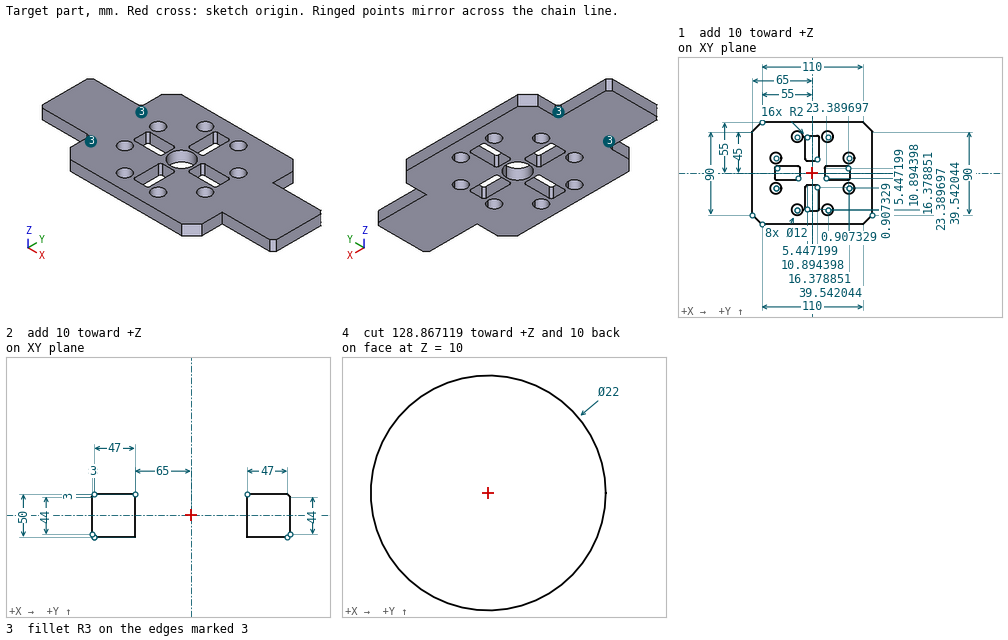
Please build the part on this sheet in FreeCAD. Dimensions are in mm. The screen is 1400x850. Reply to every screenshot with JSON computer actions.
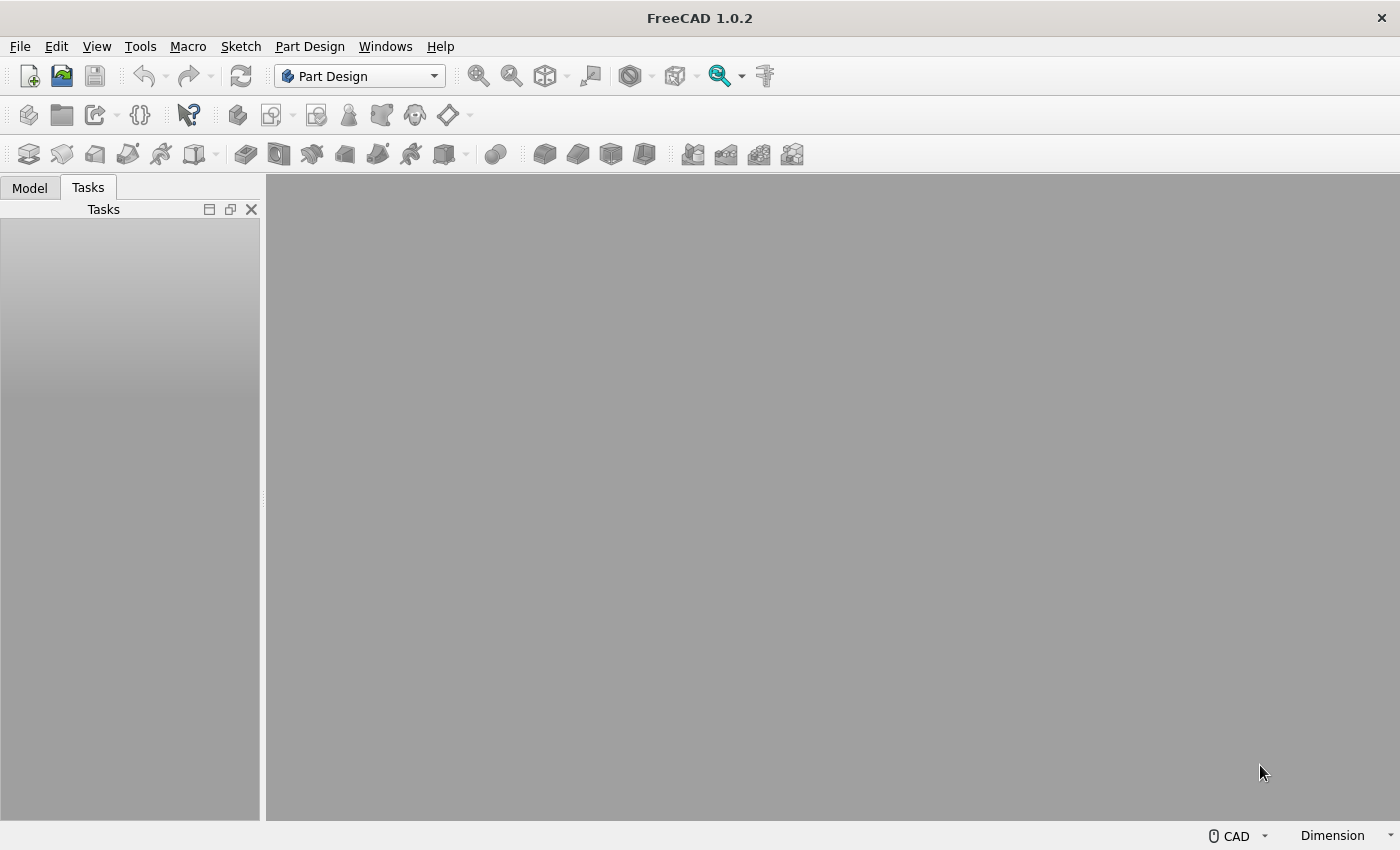
{"action": "left_click", "coordinate": [29, 76]}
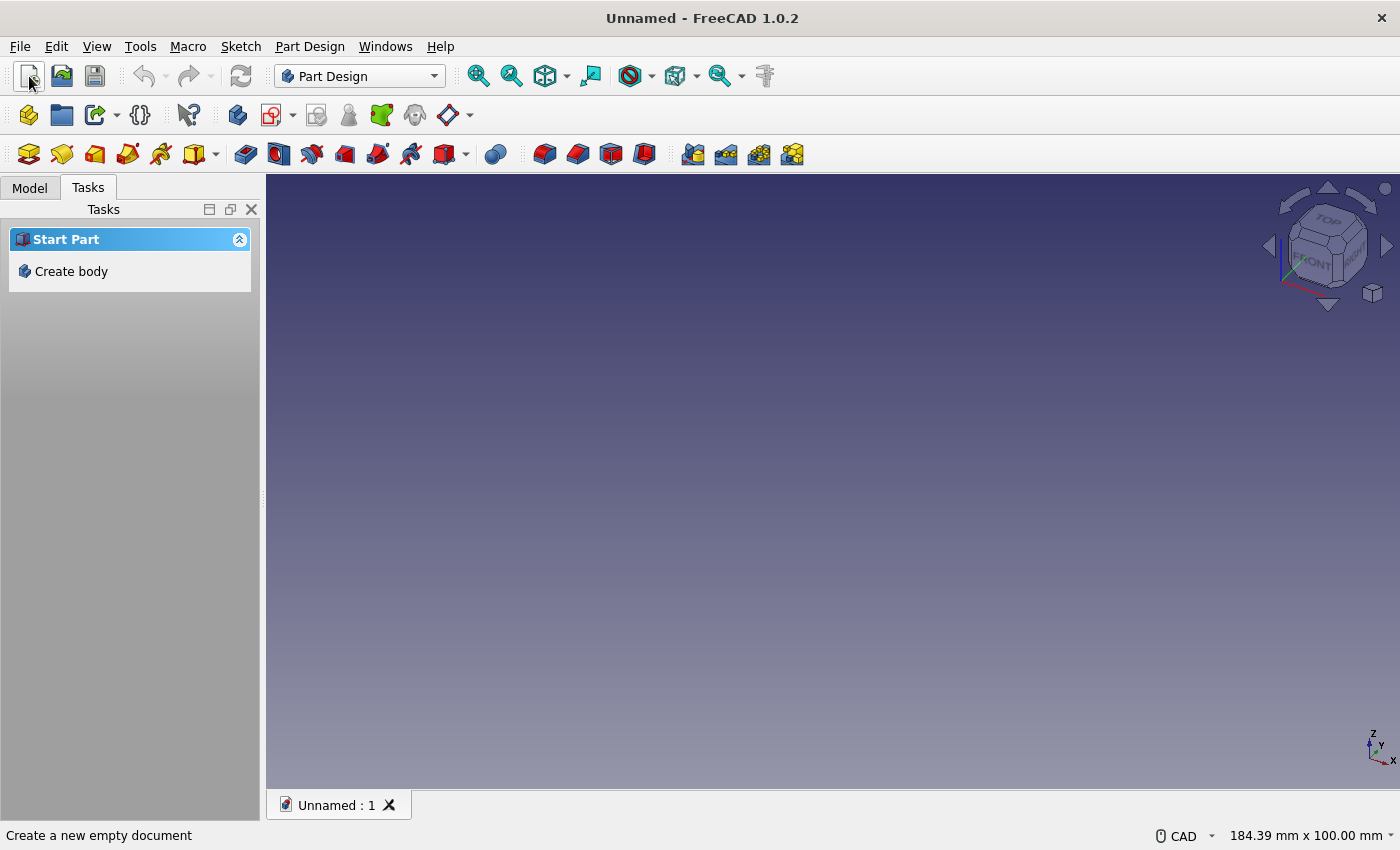
{"action": "left_click", "coordinate": [270, 116]}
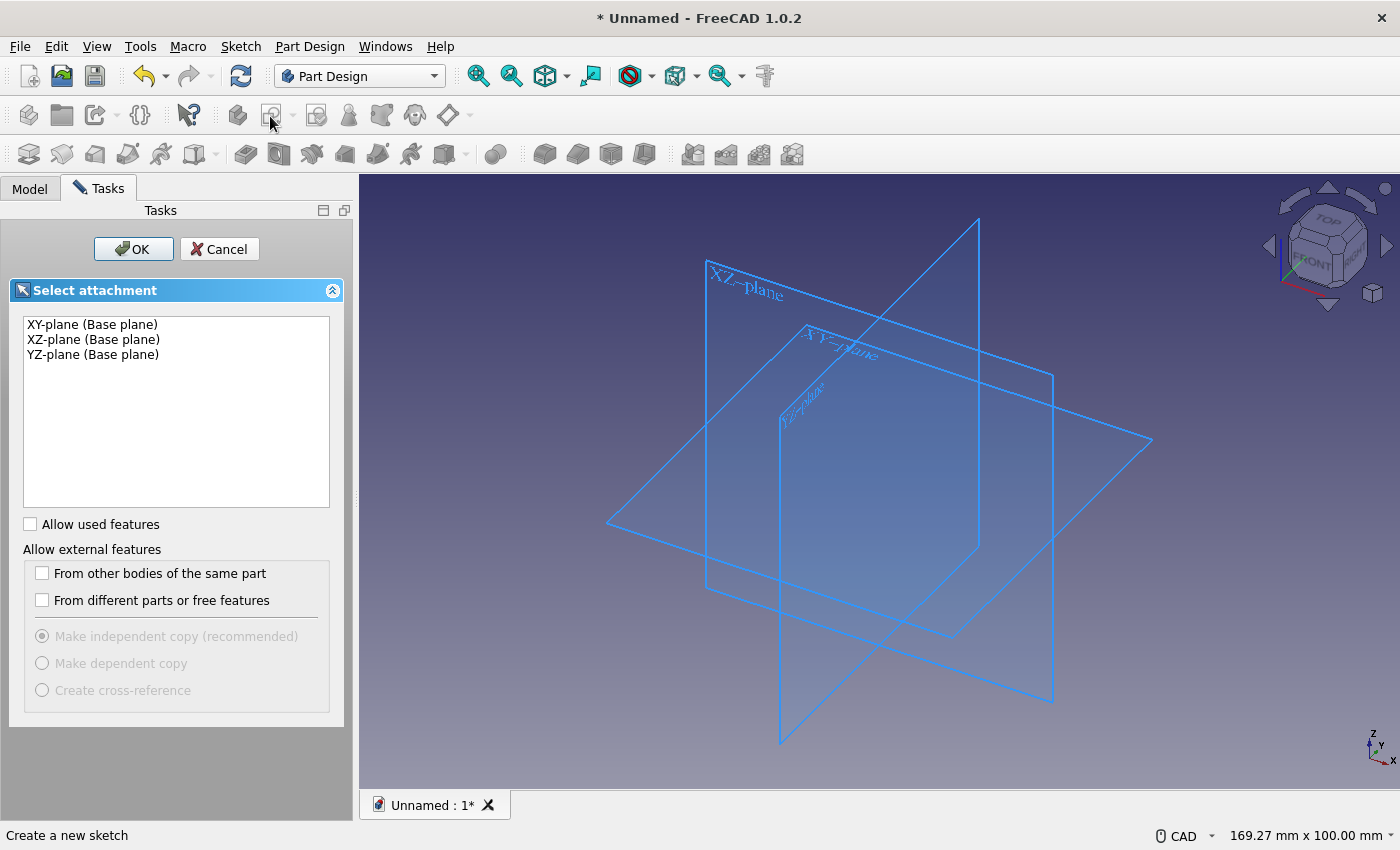
{"action": "left_click", "coordinate": [84, 324]}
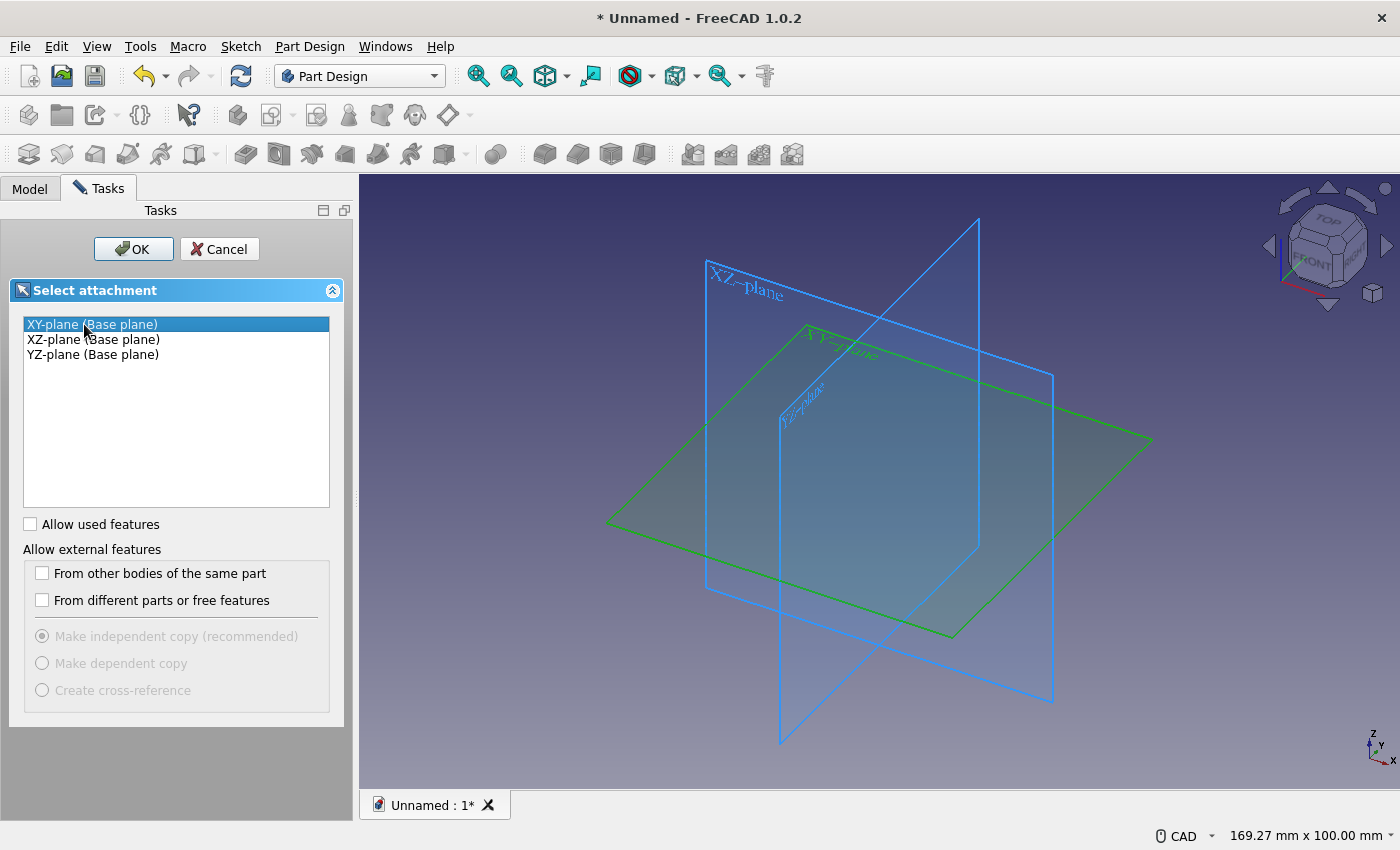
{"action": "left_click", "coordinate": [134, 249]}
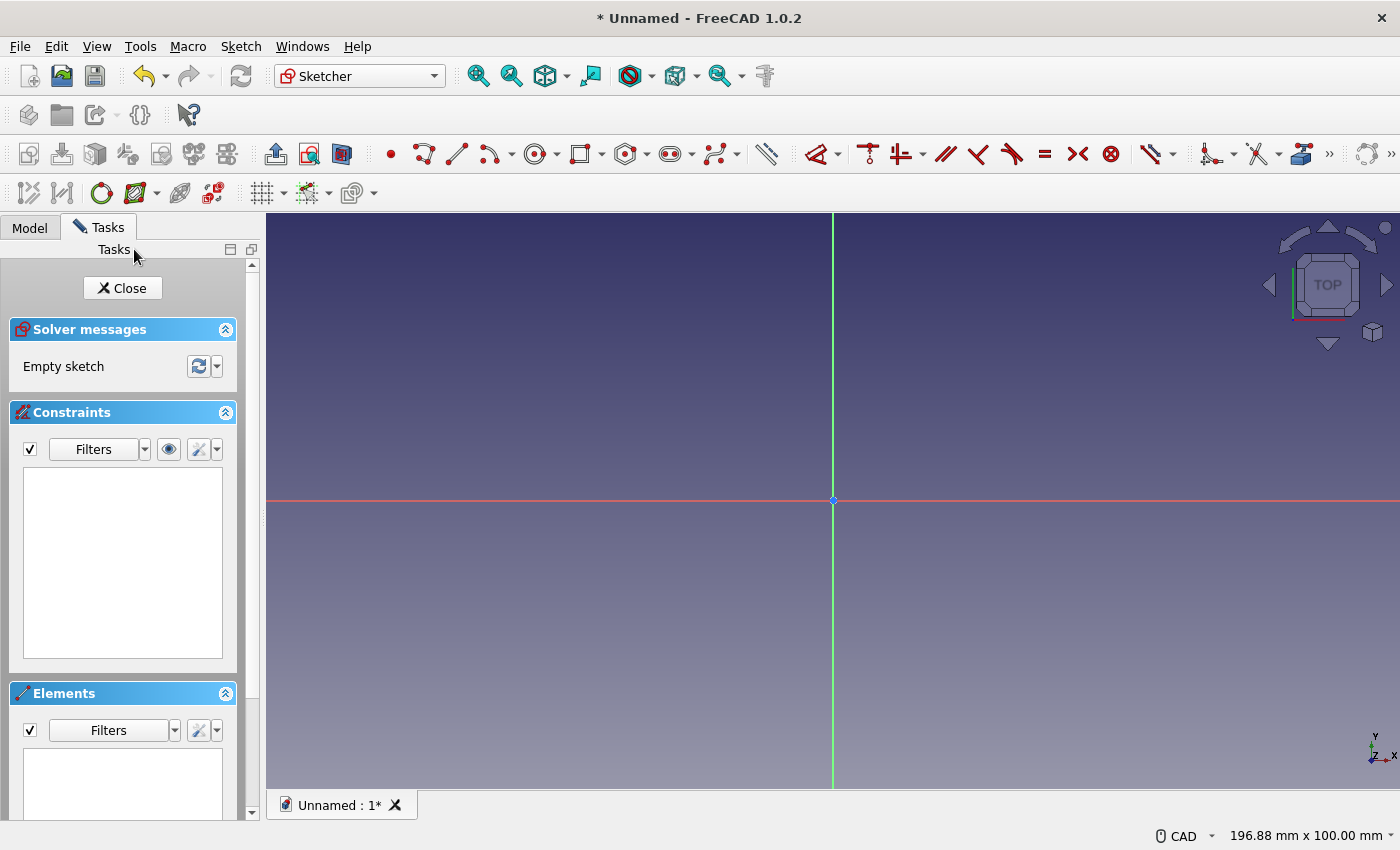
{"action": "scroll", "coordinate": [681, 501], "scroll_direction": "down", "scroll_amount": 3}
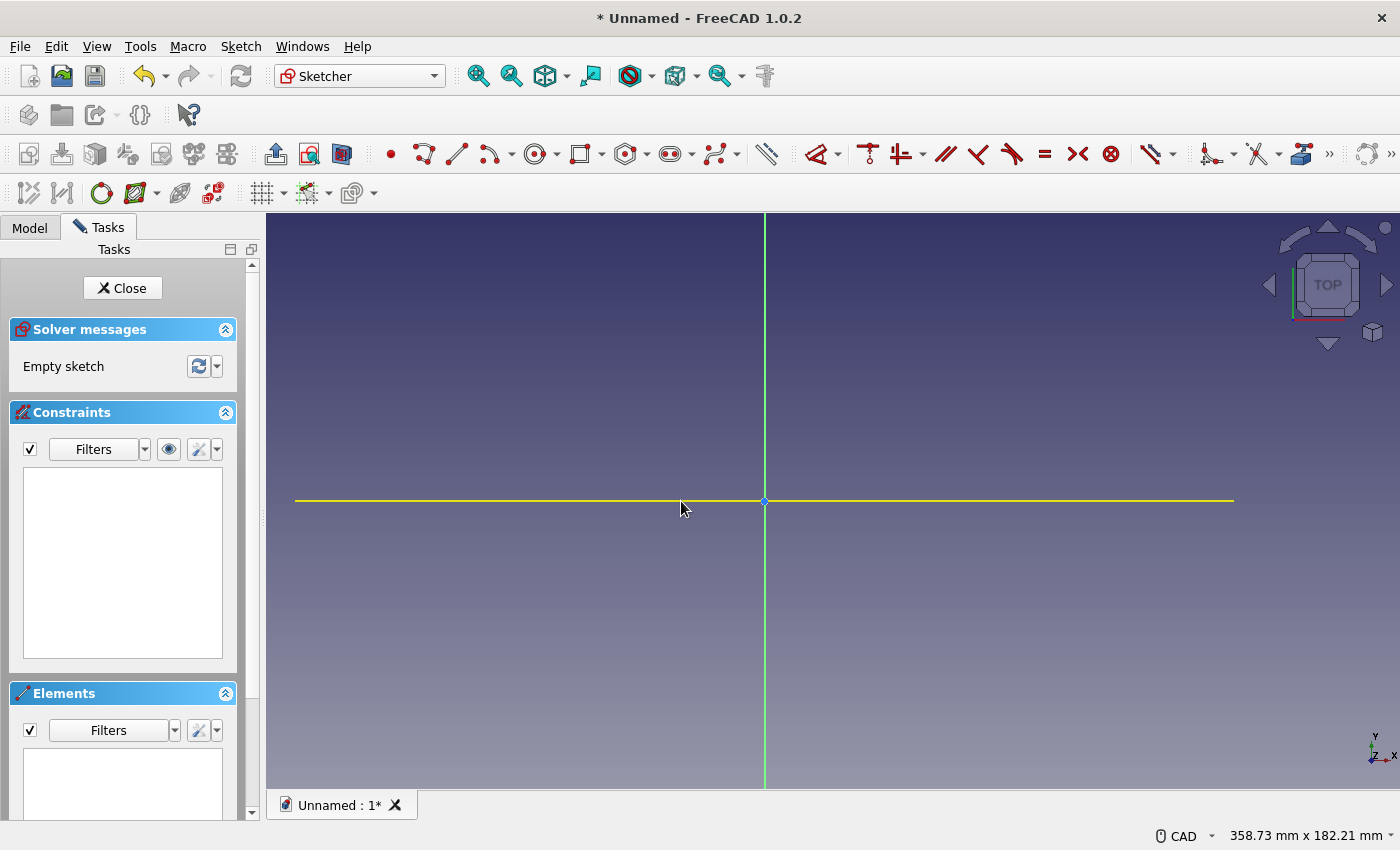
{"action": "left_click", "coordinate": [424, 154]}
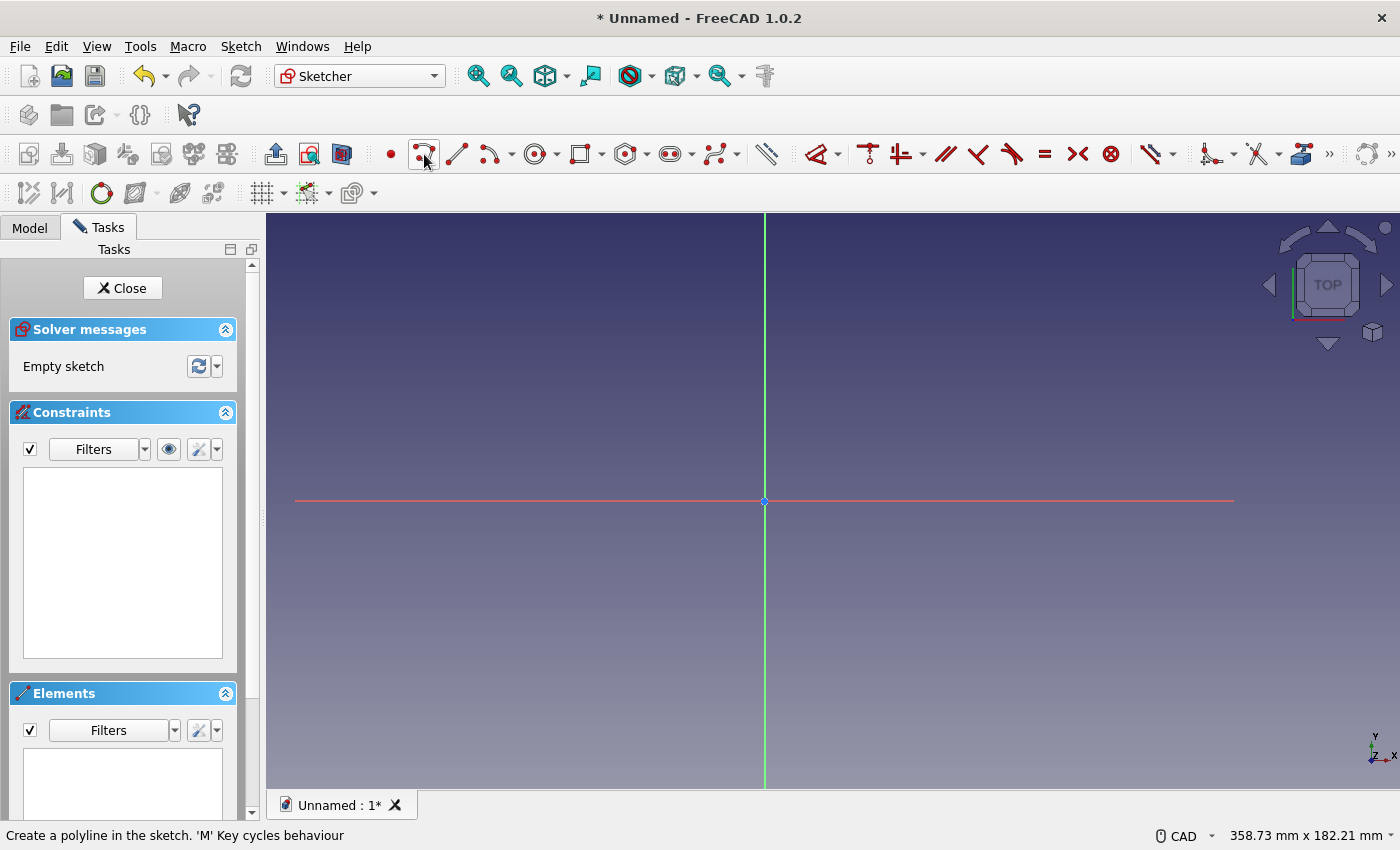
{"action": "left_click", "coordinate": [591, 327]}
{"action": "left_click", "coordinate": [559, 359]}
{"action": "left_click", "coordinate": [559, 643]}
{"action": "left_click", "coordinate": [591, 675]}
{"action": "left_click", "coordinate": [938, 675]}
{"action": "left_click", "coordinate": [970, 643]}
{"action": "left_click", "coordinate": [970, 359]}
{"action": "left_click", "coordinate": [938, 327]}
{"action": "left_click", "coordinate": [591, 328]}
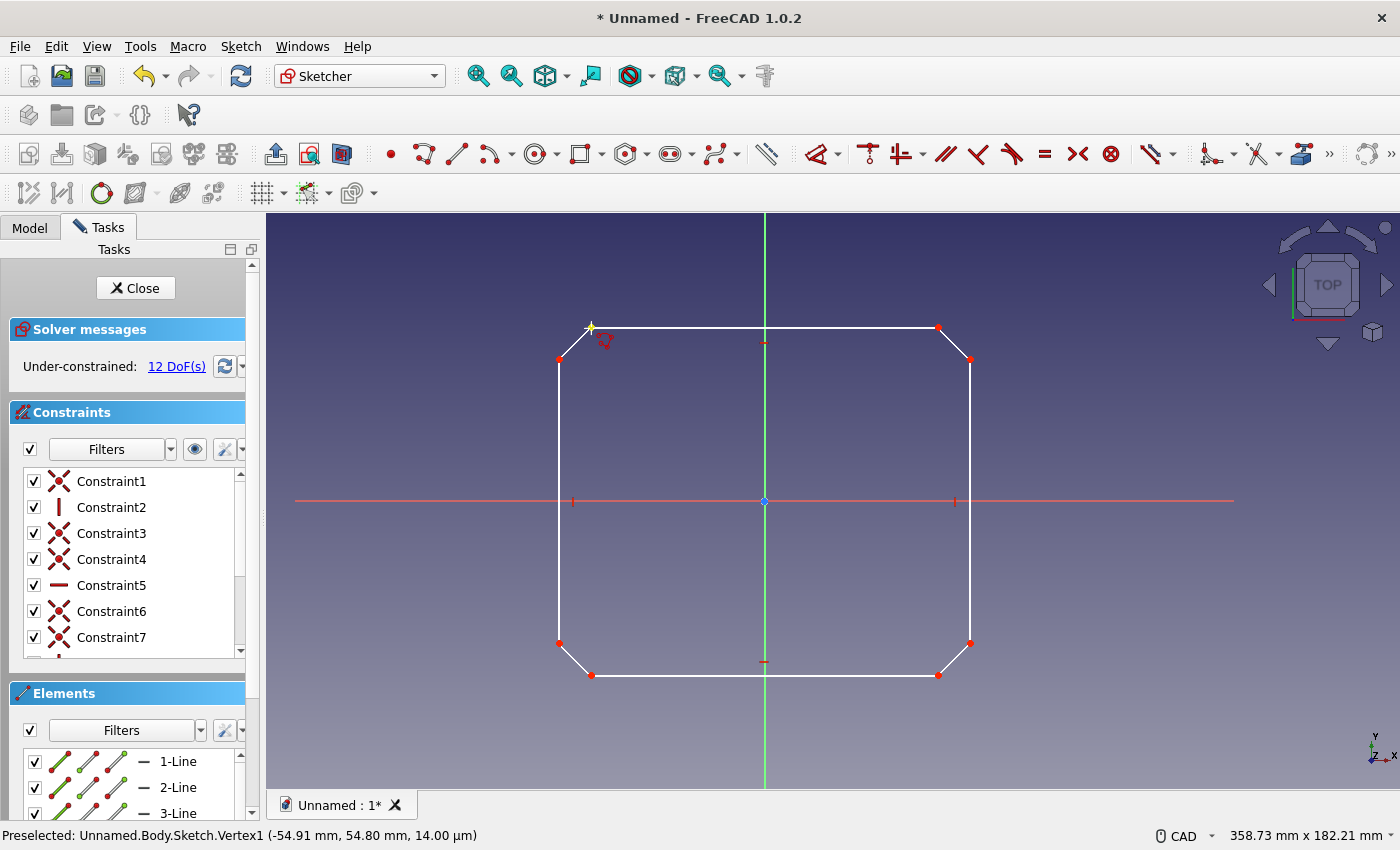
{"action": "left_click", "coordinate": [457, 154]}